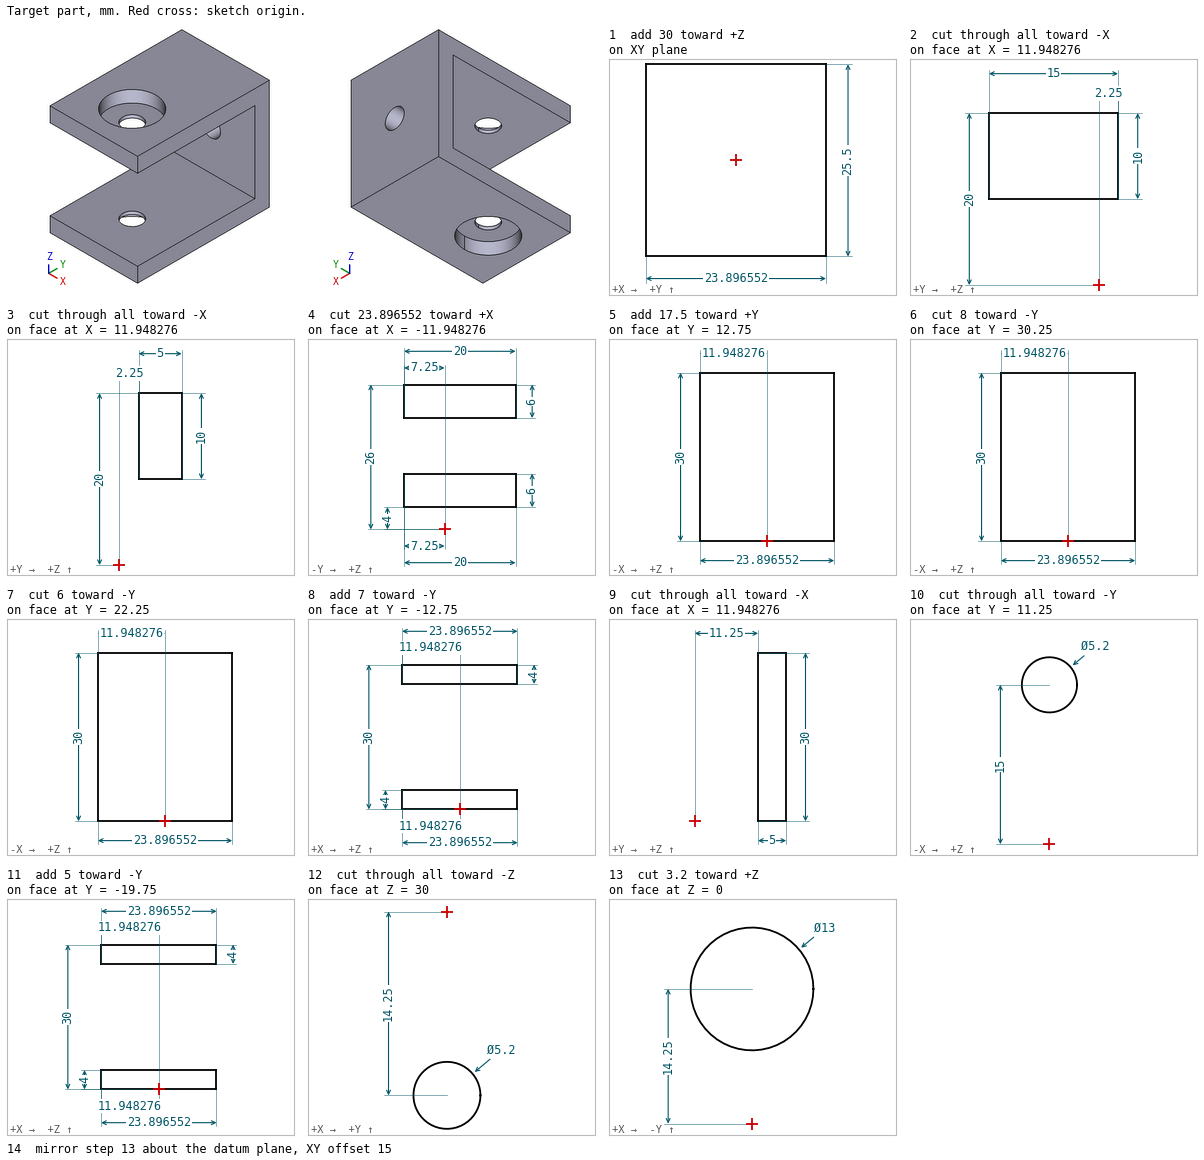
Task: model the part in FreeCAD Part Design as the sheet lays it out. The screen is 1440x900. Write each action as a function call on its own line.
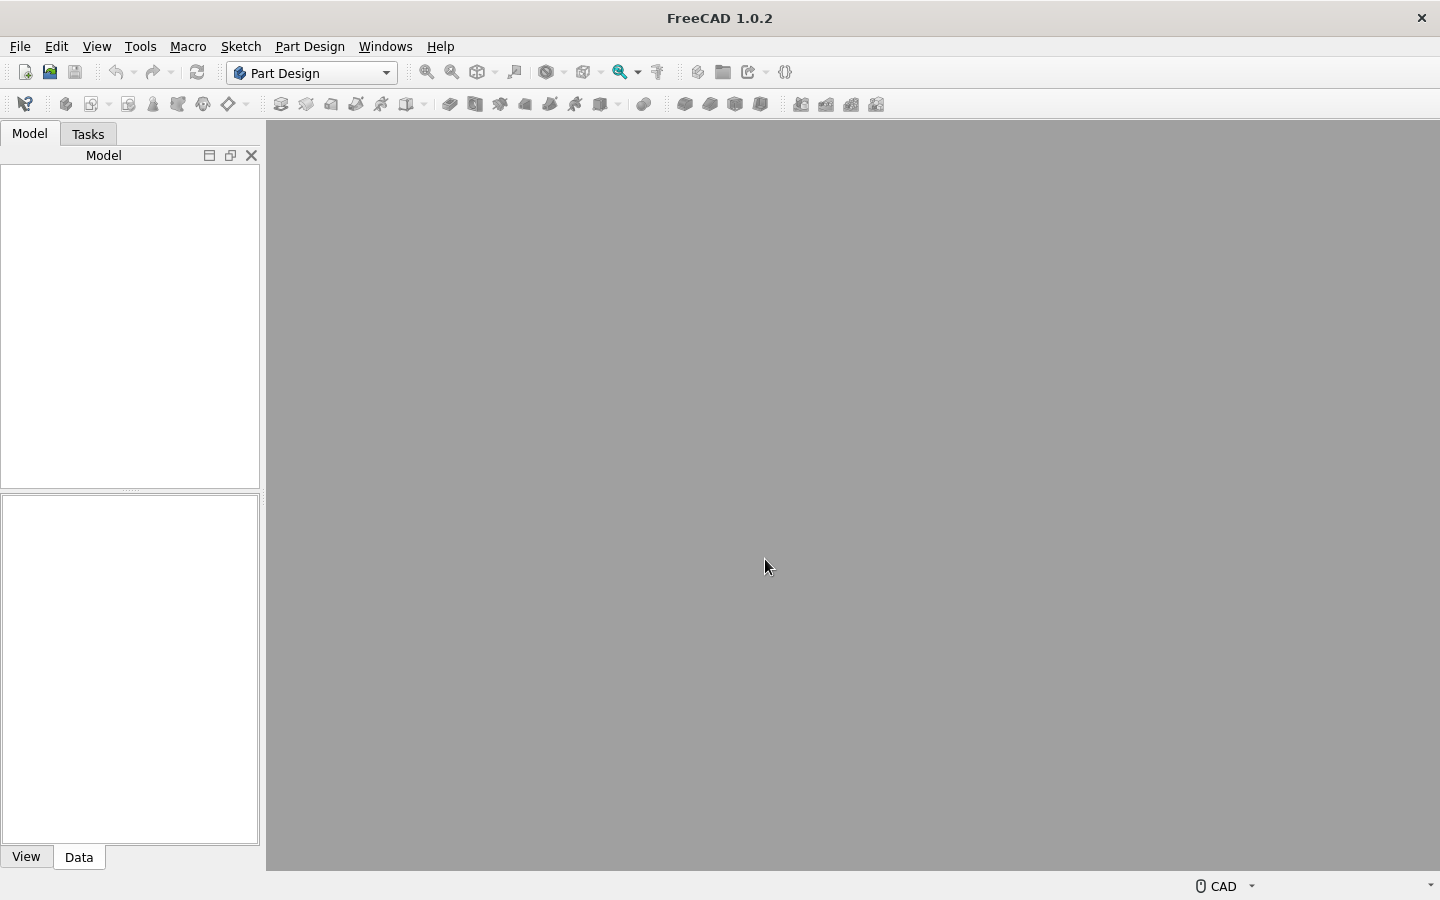
key(ctrl+n)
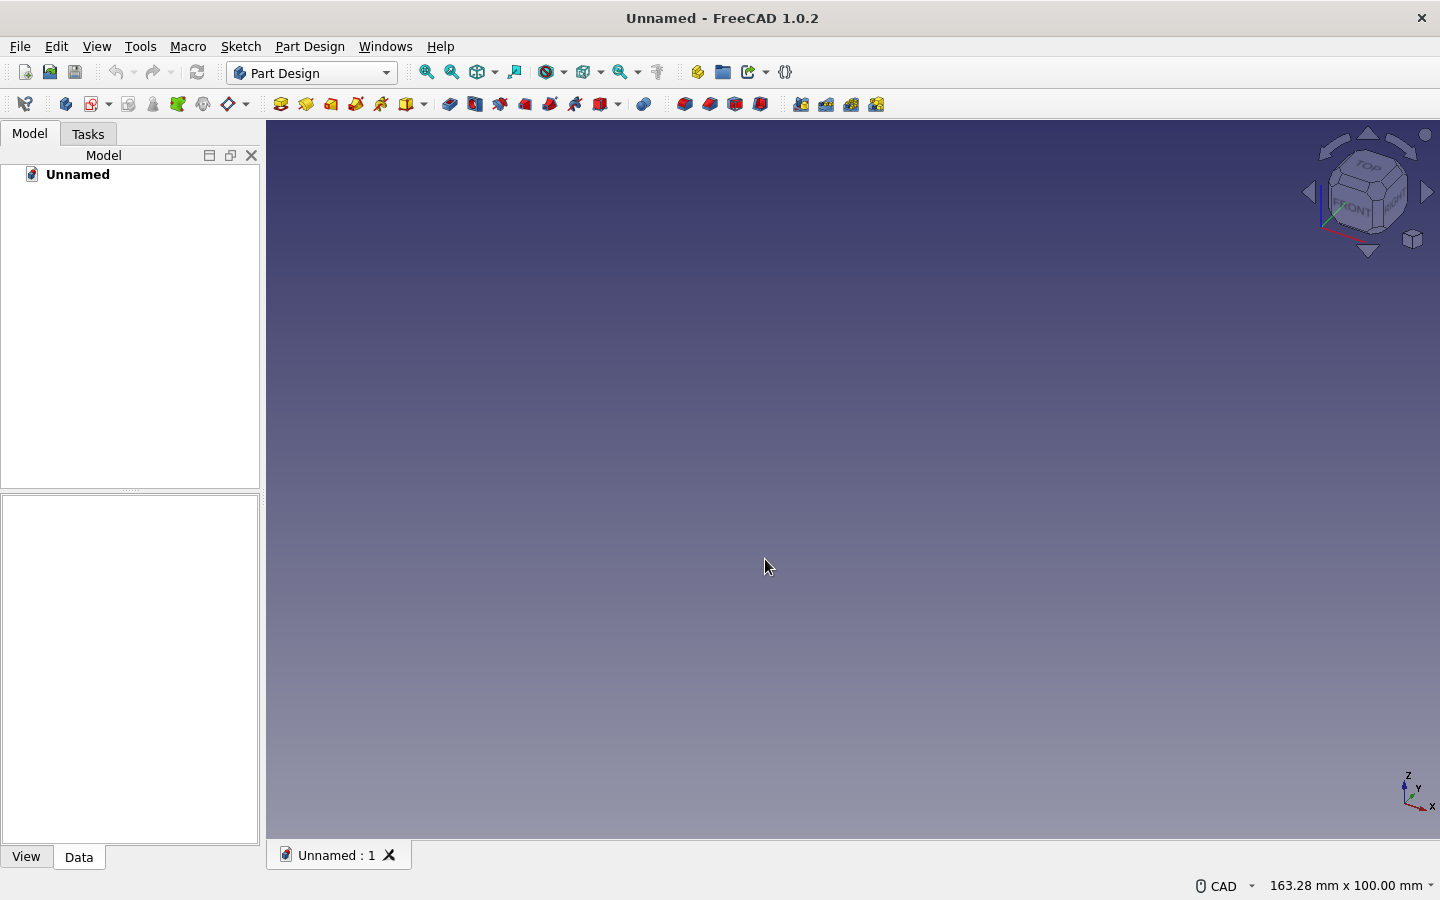
click(90, 104)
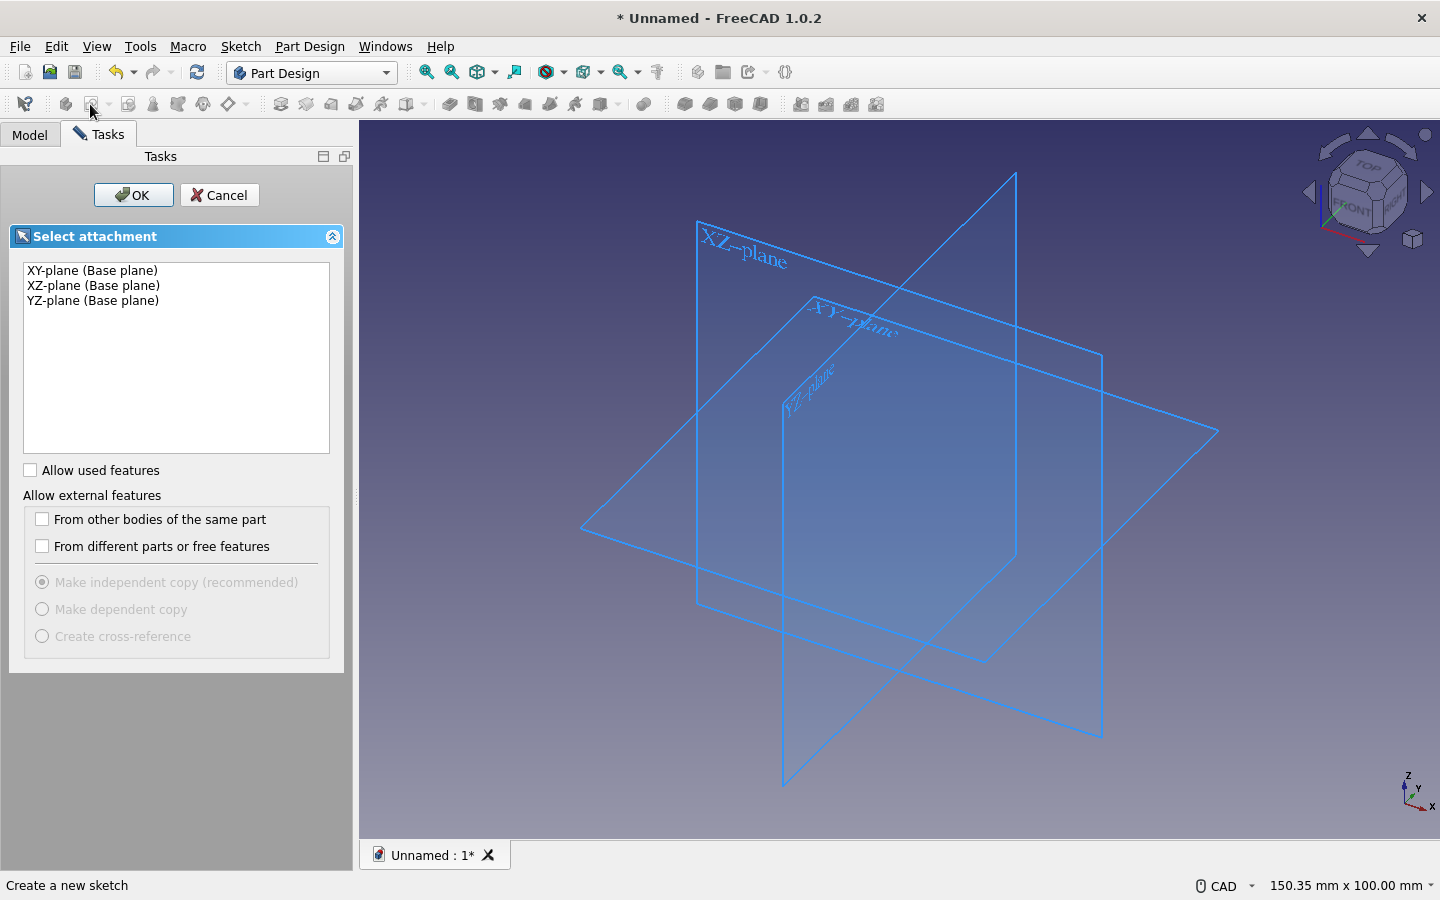
click(84, 270)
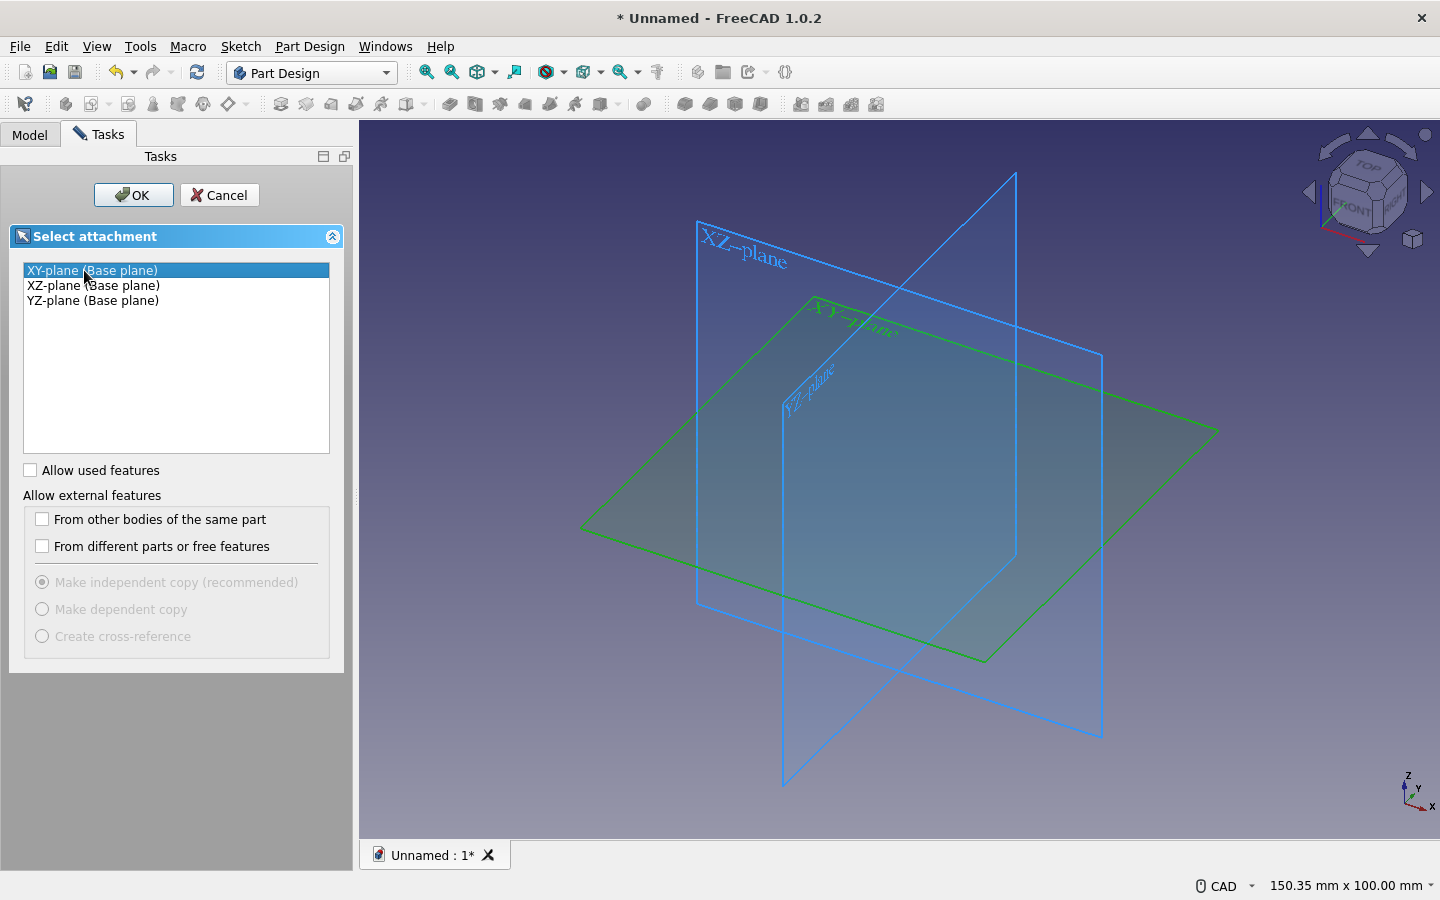
click(134, 195)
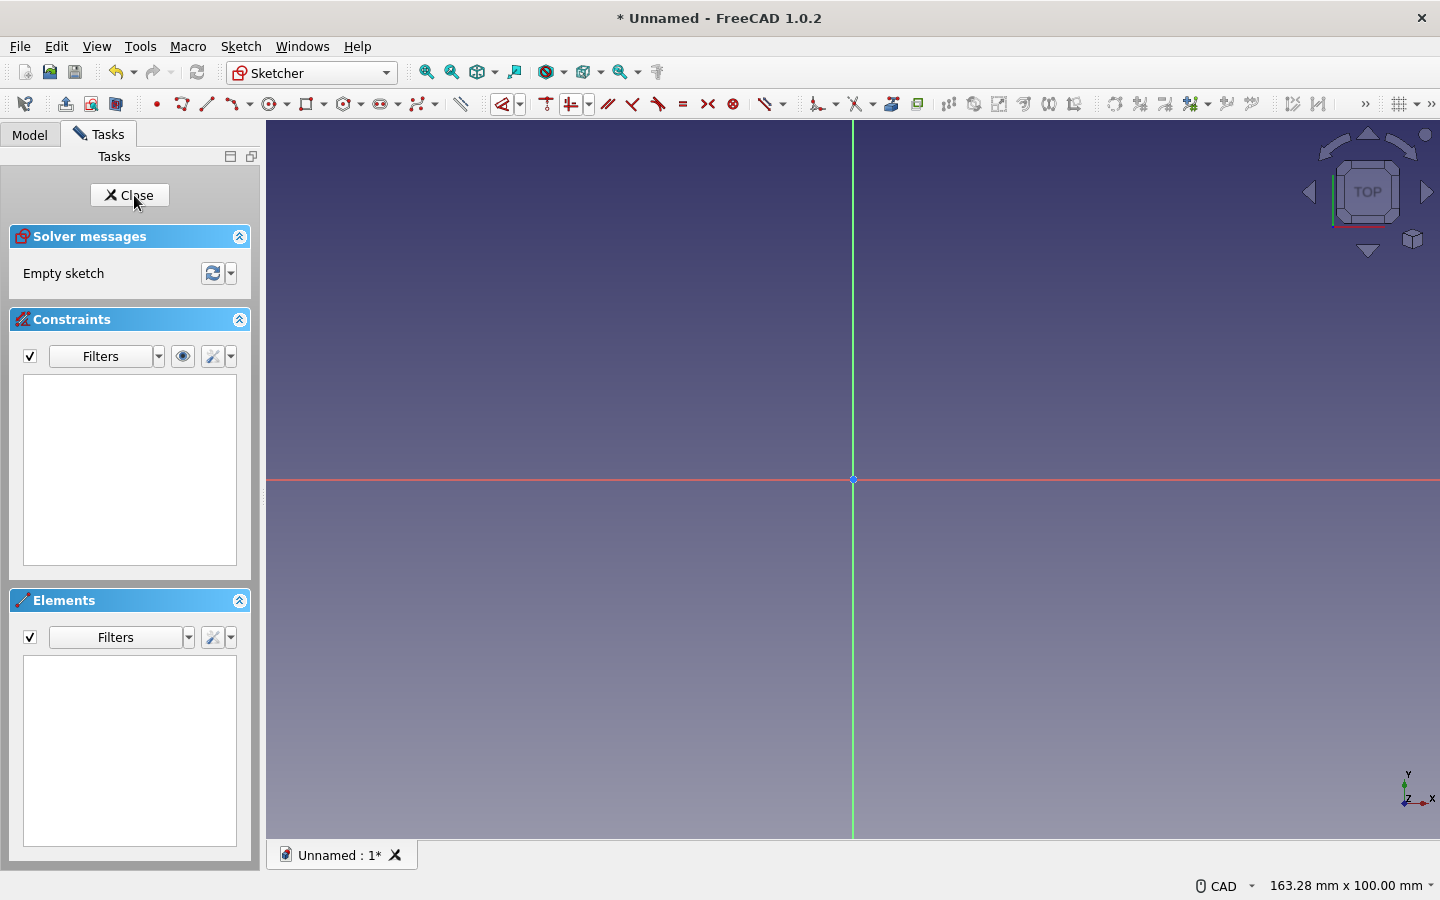
scroll(893, 480, up, 5)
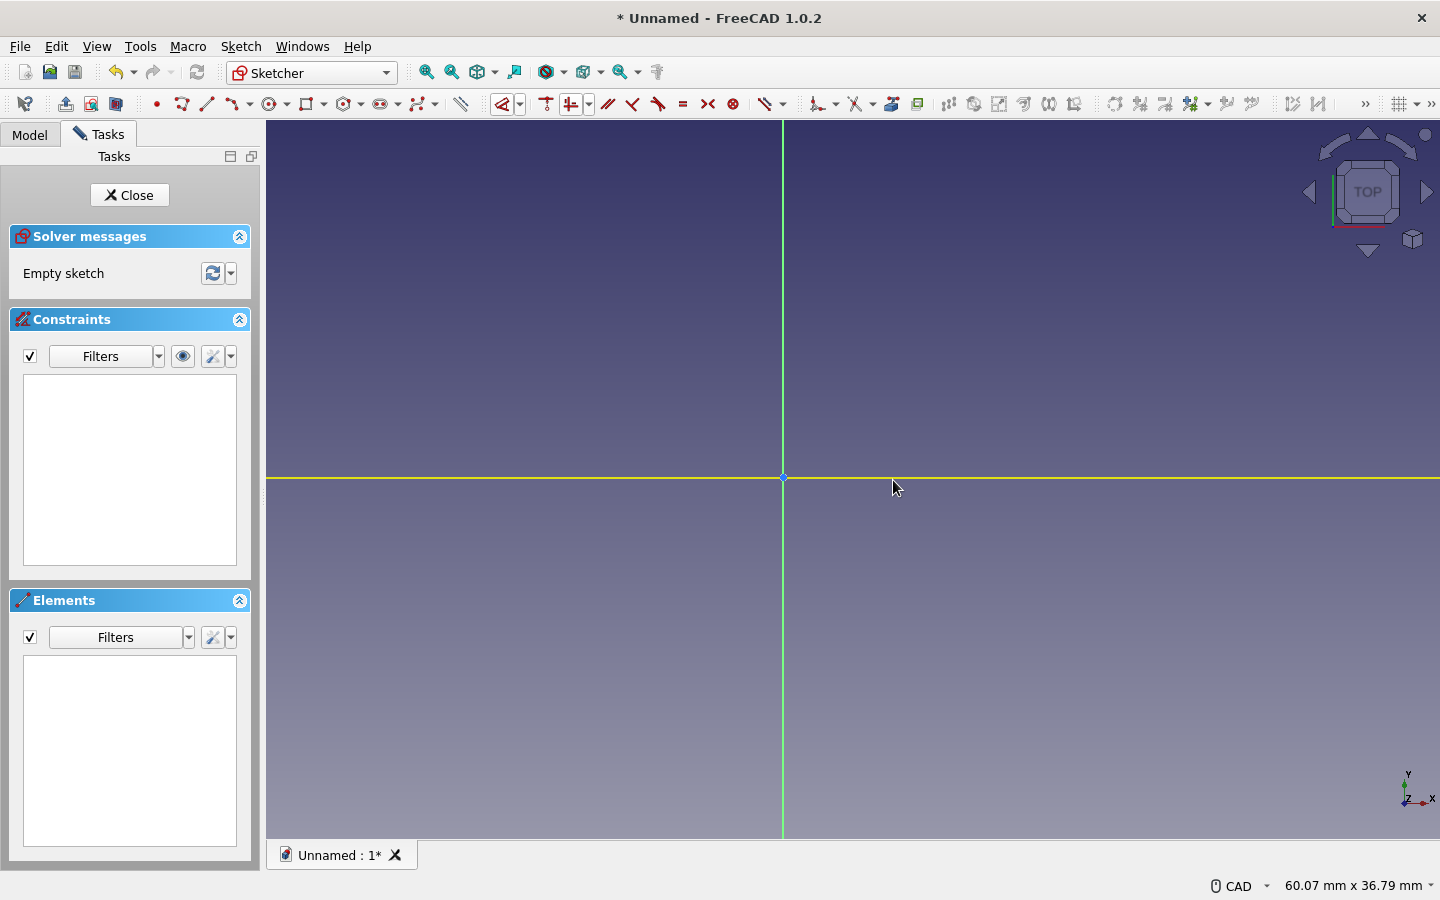
key(g)
key(v)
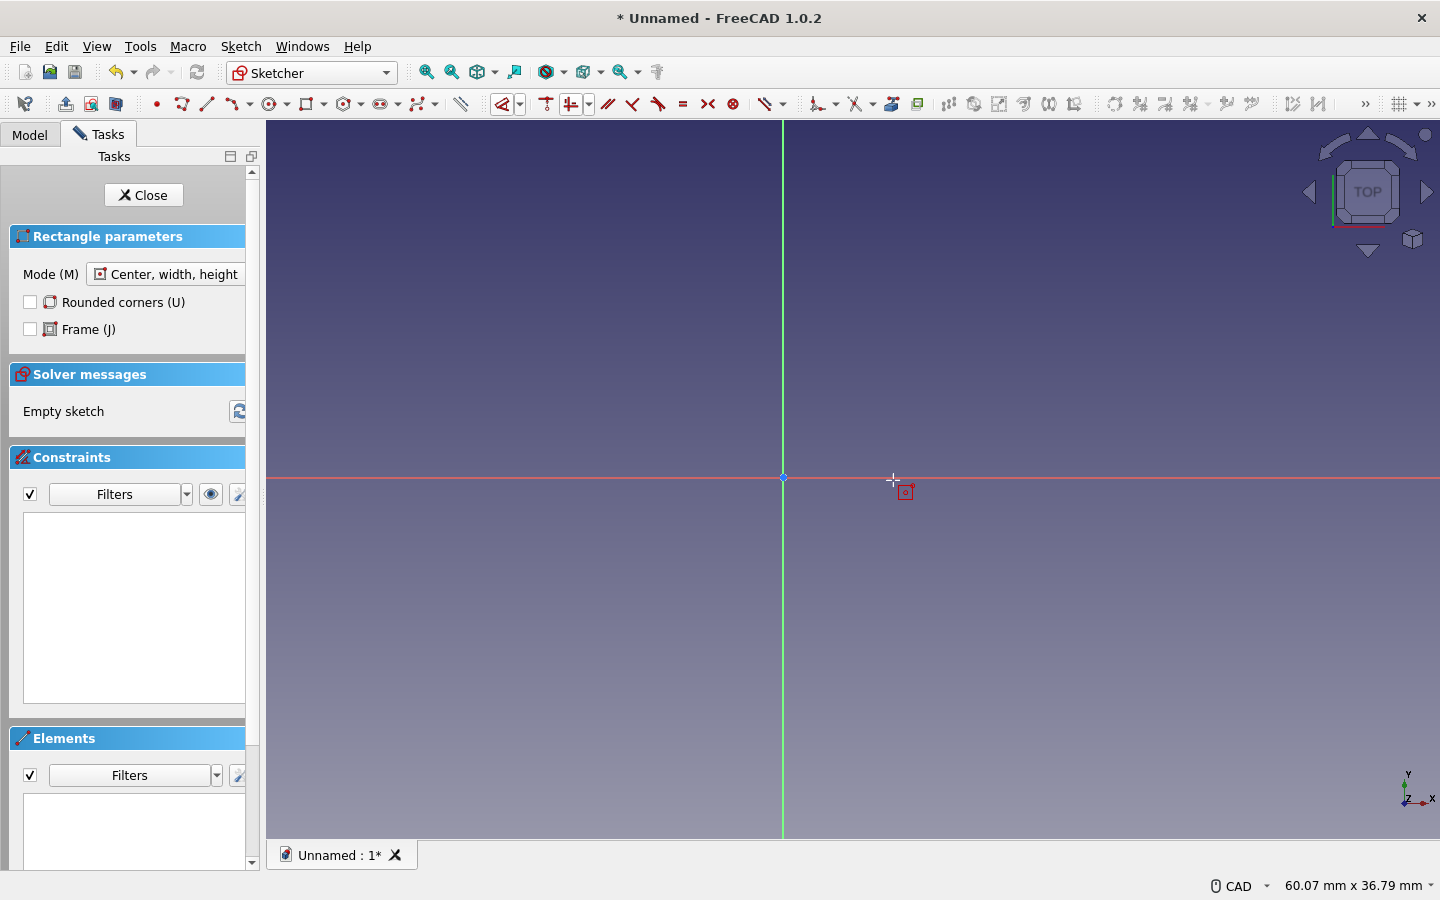
click(783, 478)
move(1017, 229)